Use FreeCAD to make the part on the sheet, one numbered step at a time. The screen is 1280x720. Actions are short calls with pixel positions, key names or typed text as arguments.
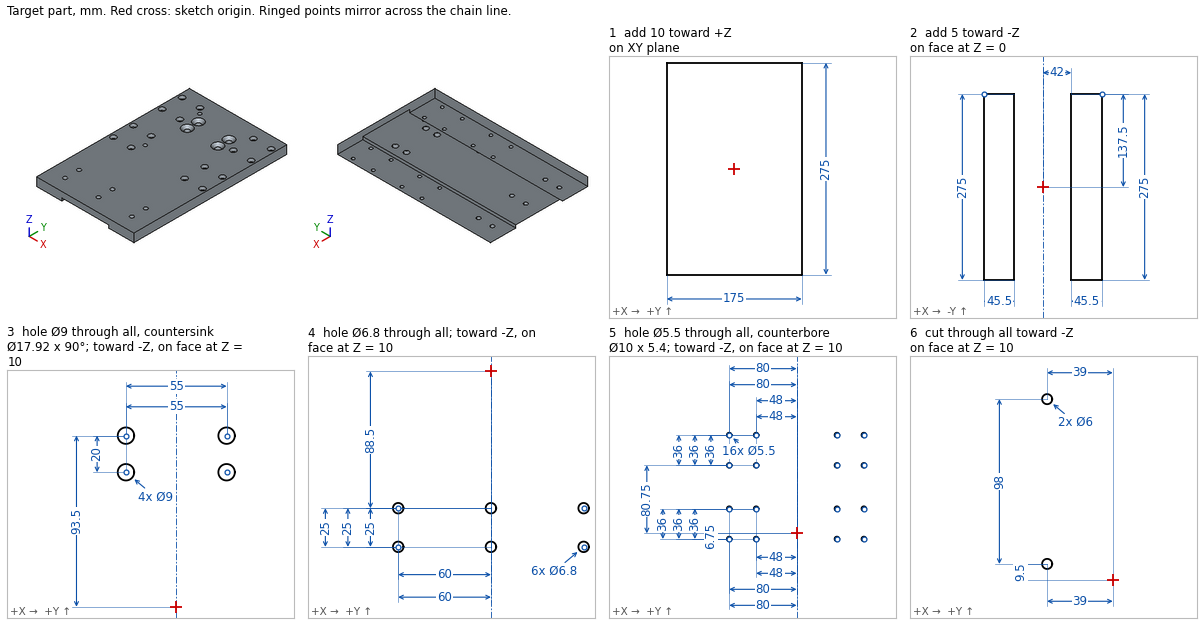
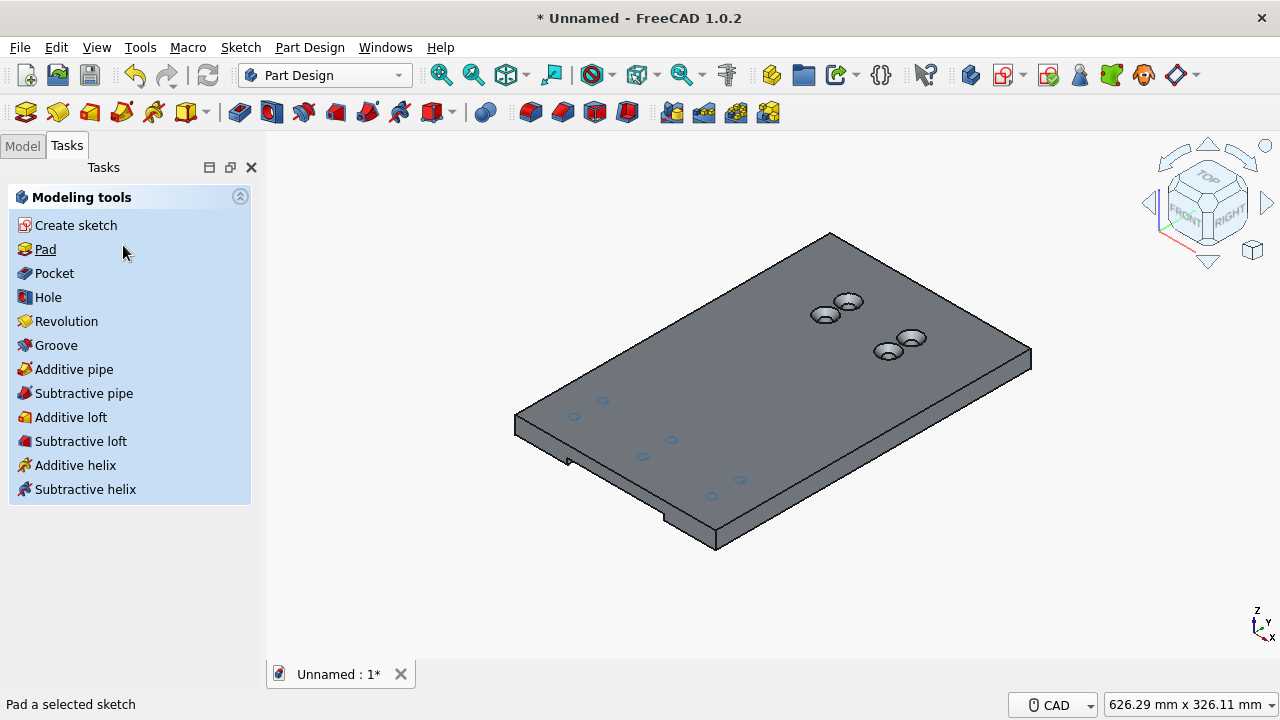
click(272, 112)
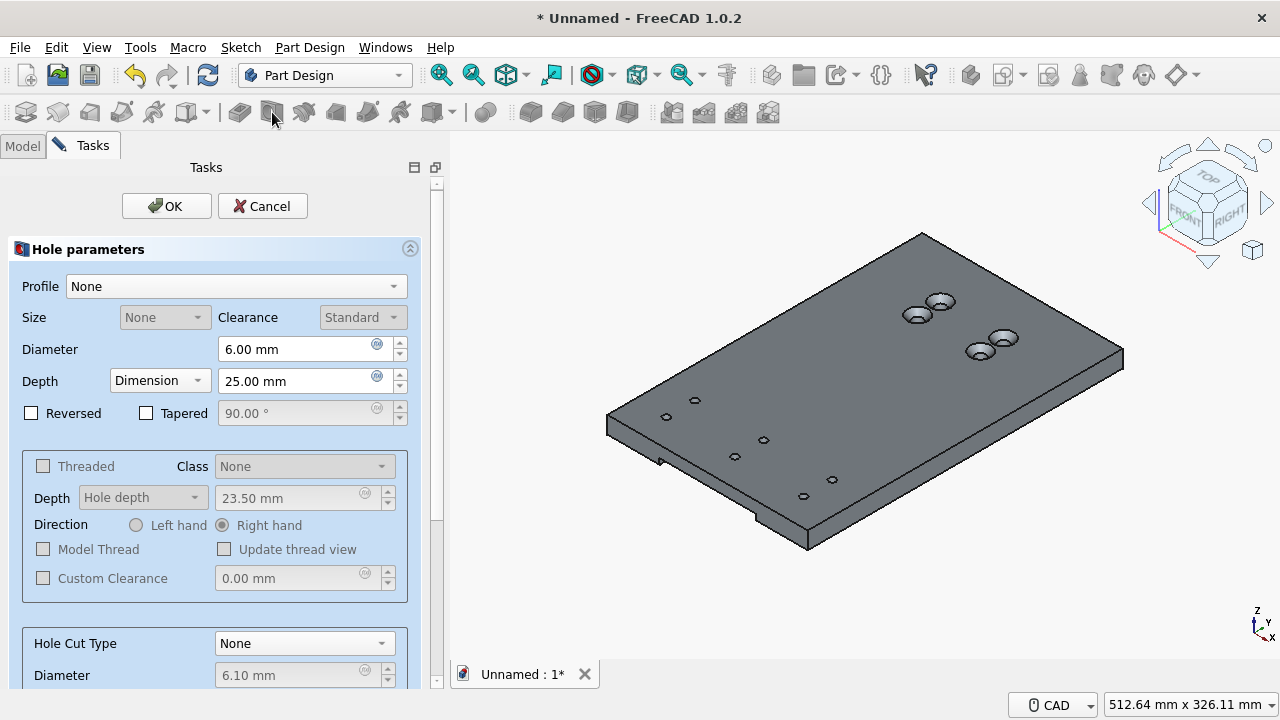
triple_click(305, 349)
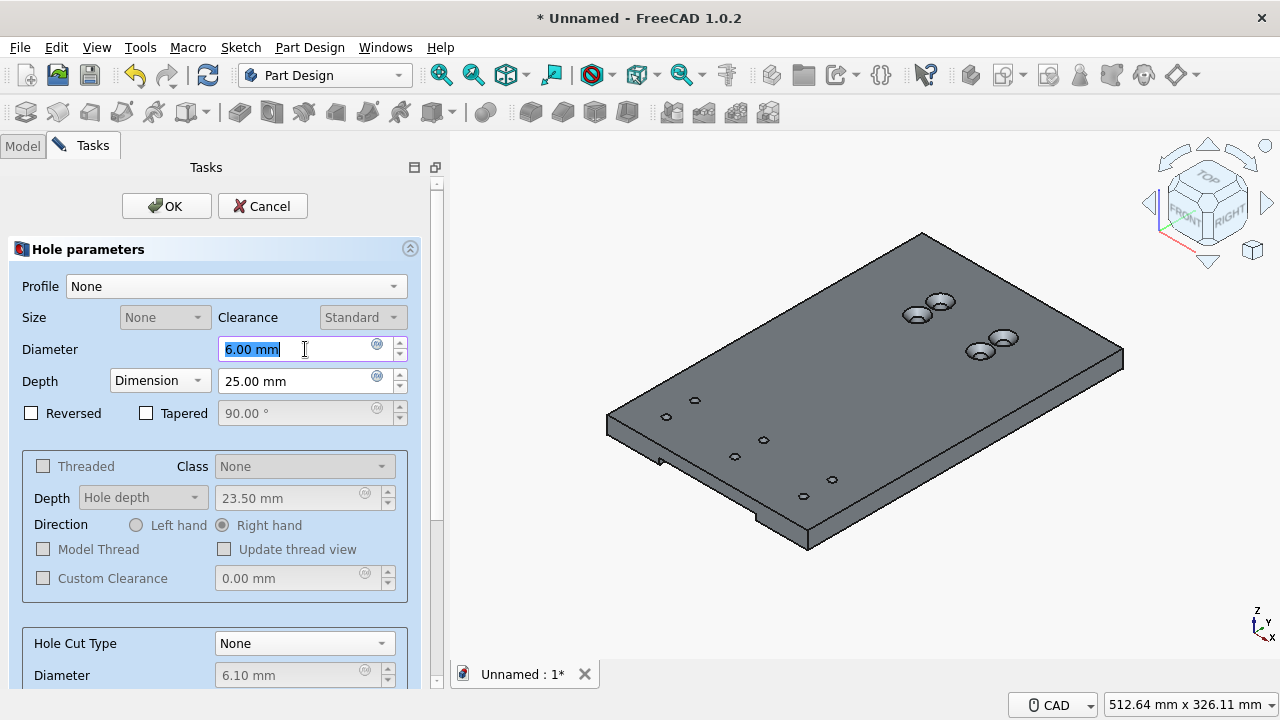
text(6.8)
key(Tab)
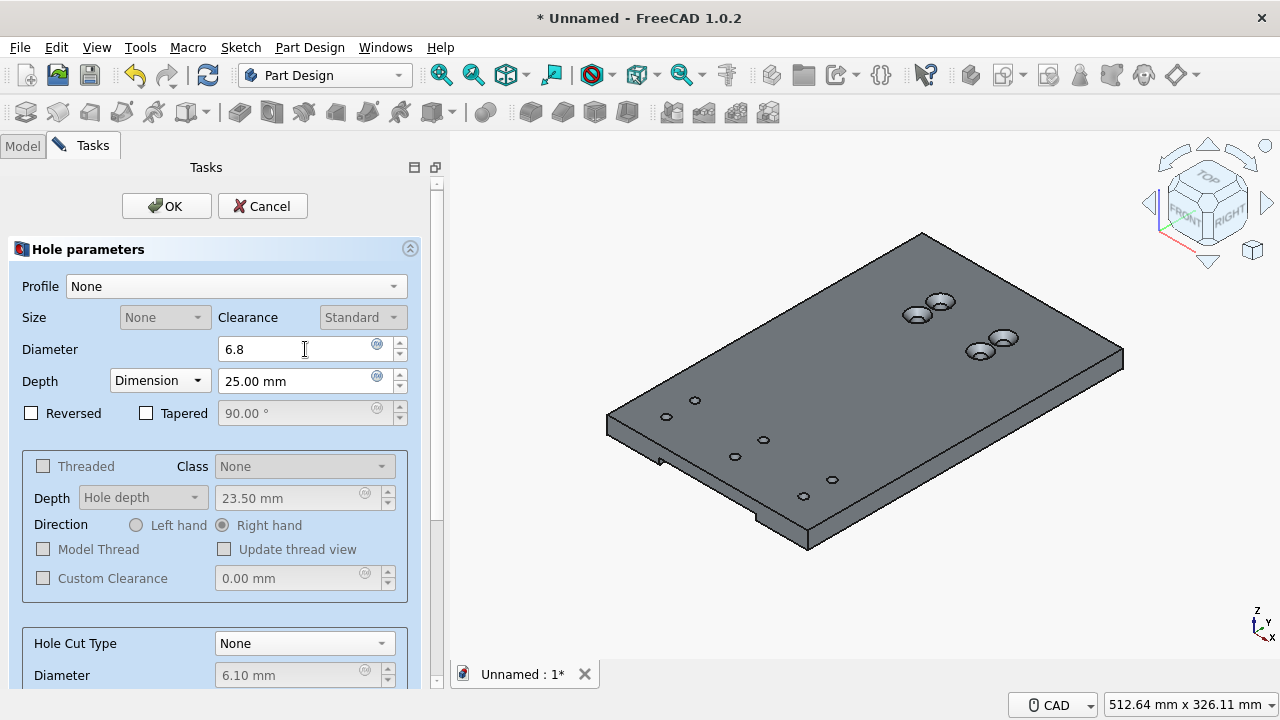
click(161, 380)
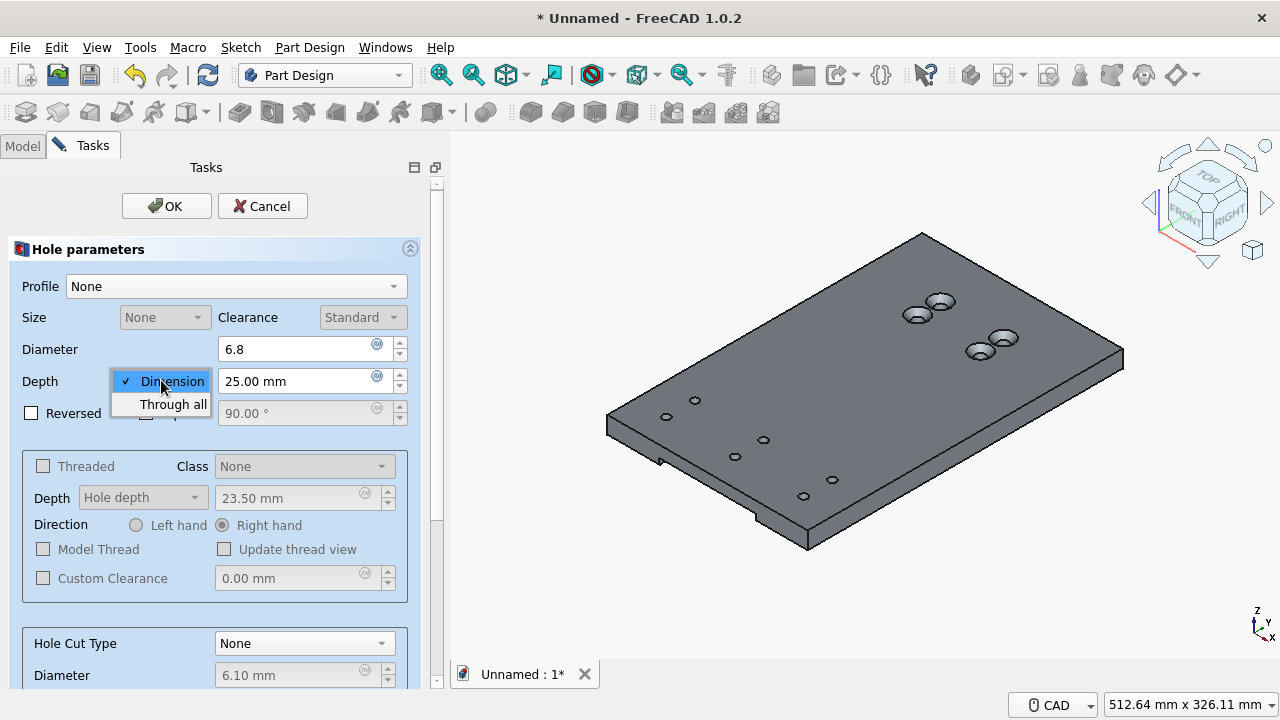
click(160, 404)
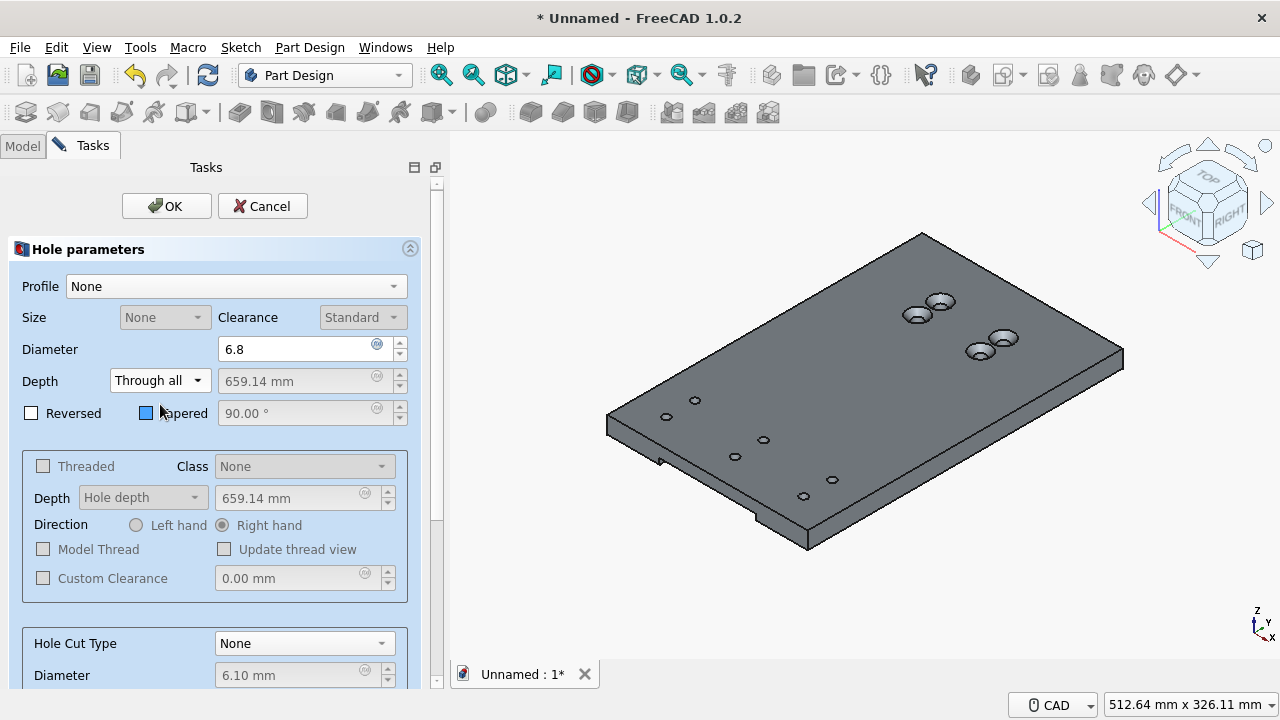
click(167, 206)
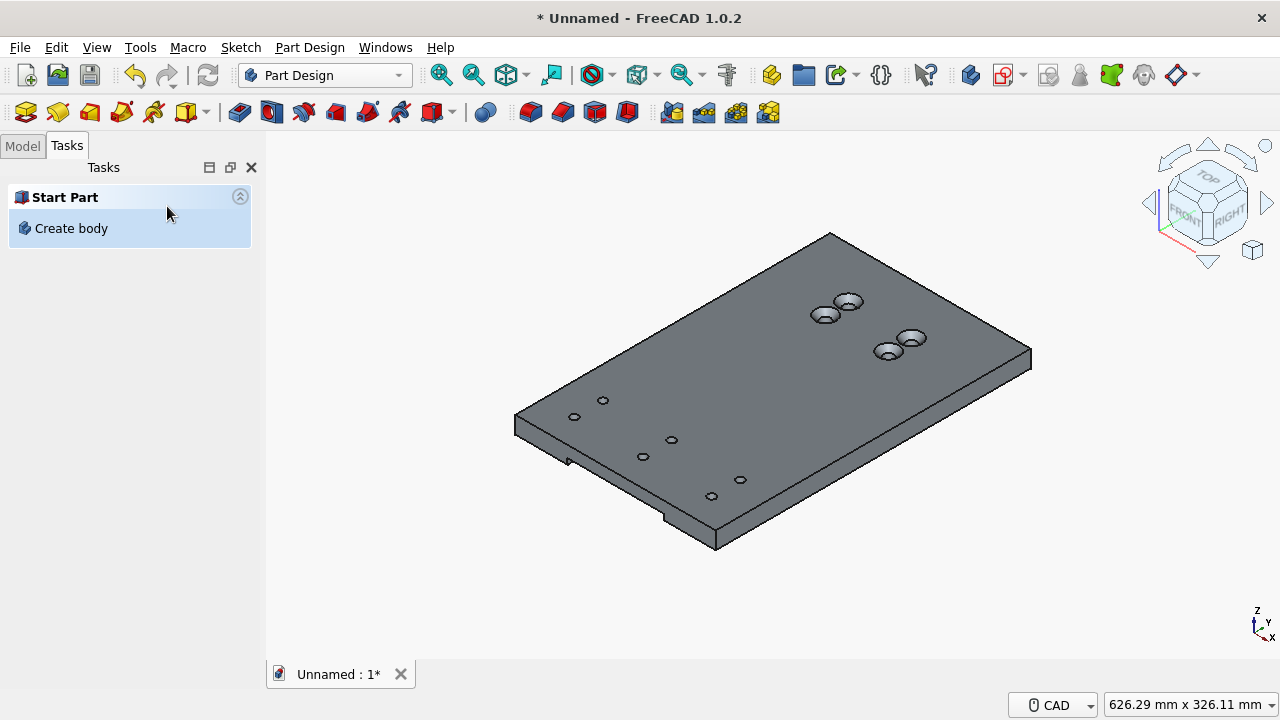
click(773, 381)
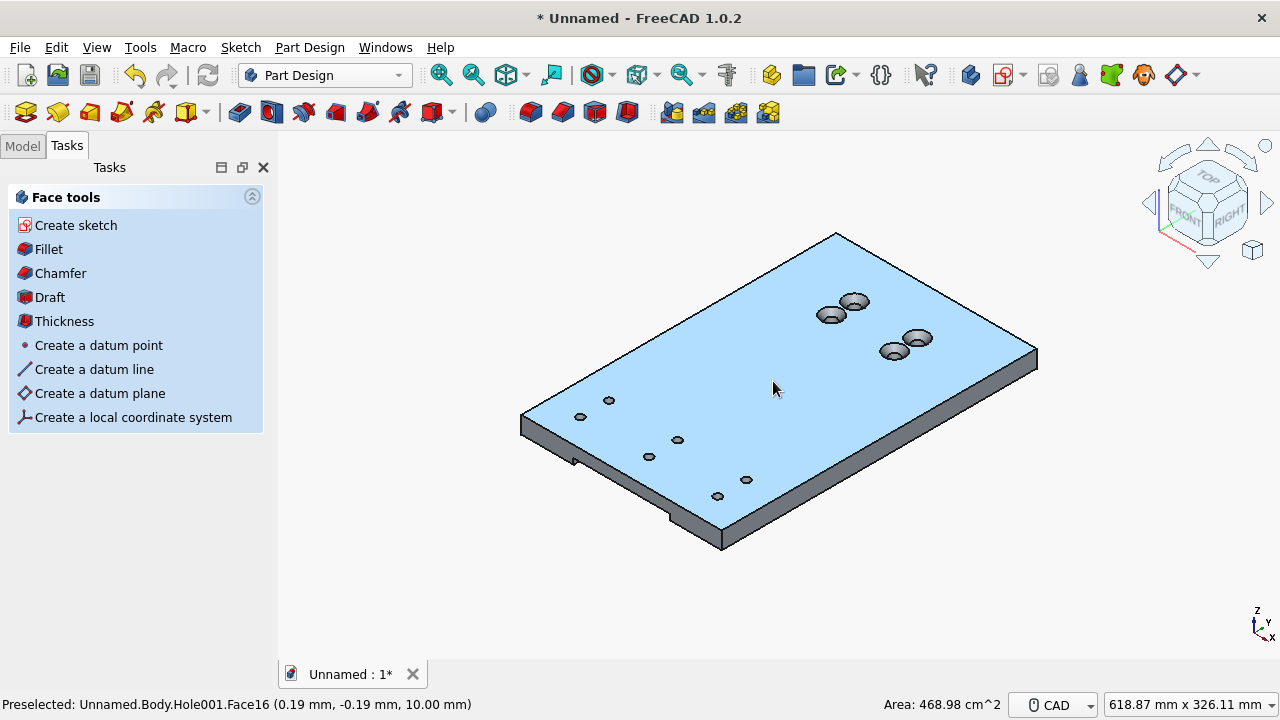
click(1004, 76)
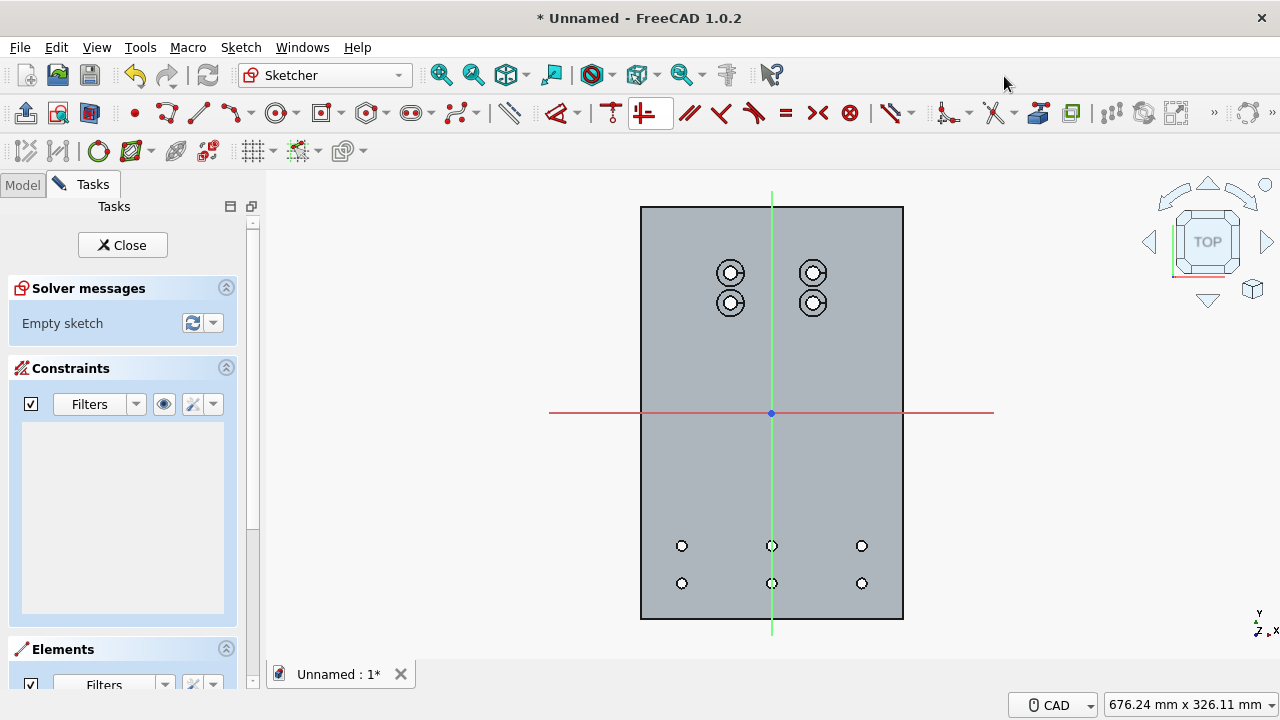
scroll(908, 198, up, 2)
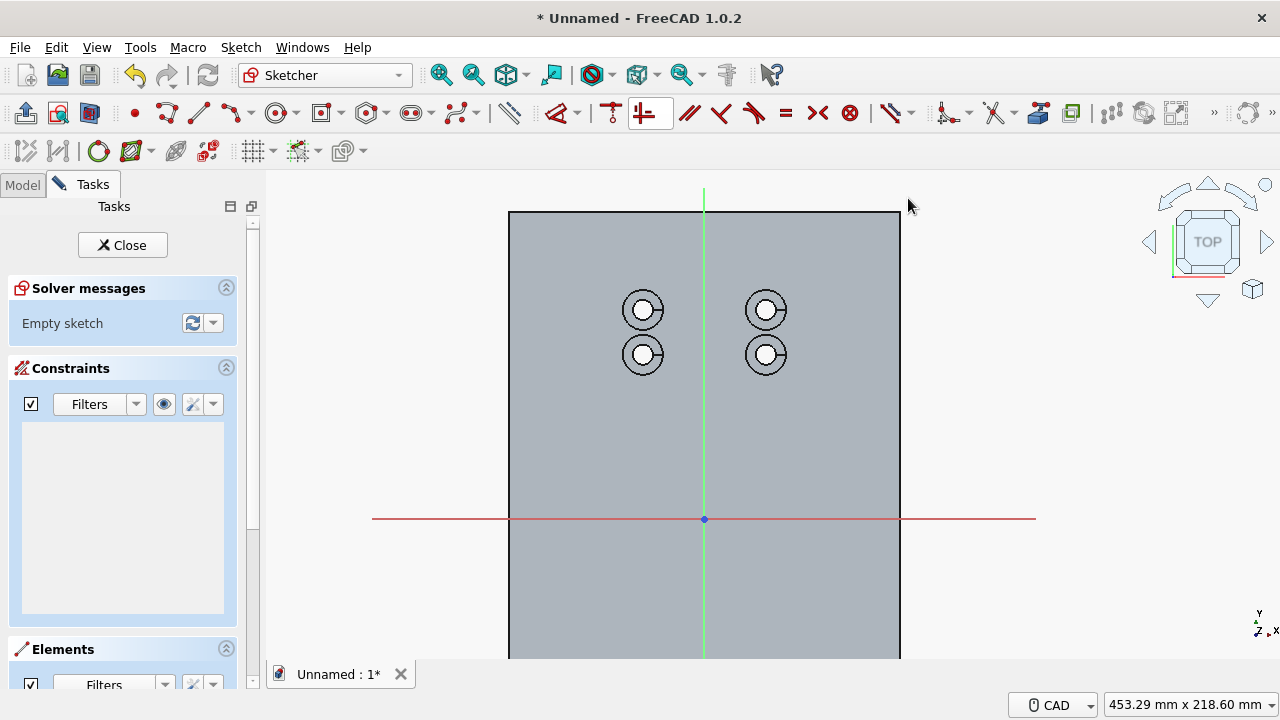
key(g)
key(c)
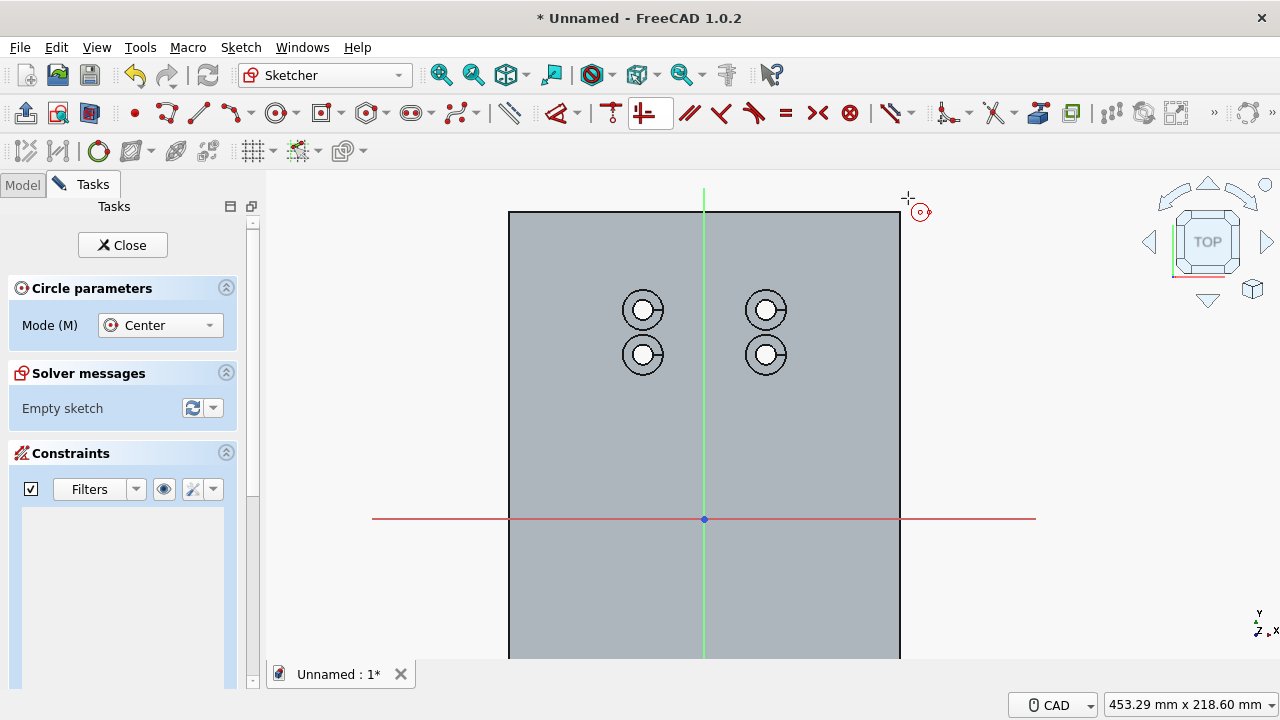
scroll(525, 258, up, 7)